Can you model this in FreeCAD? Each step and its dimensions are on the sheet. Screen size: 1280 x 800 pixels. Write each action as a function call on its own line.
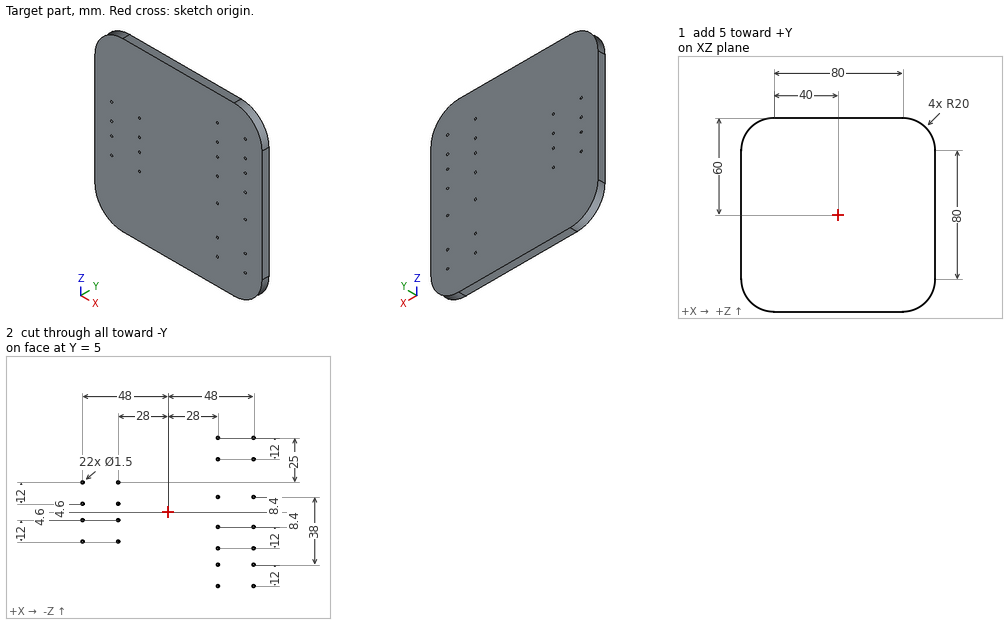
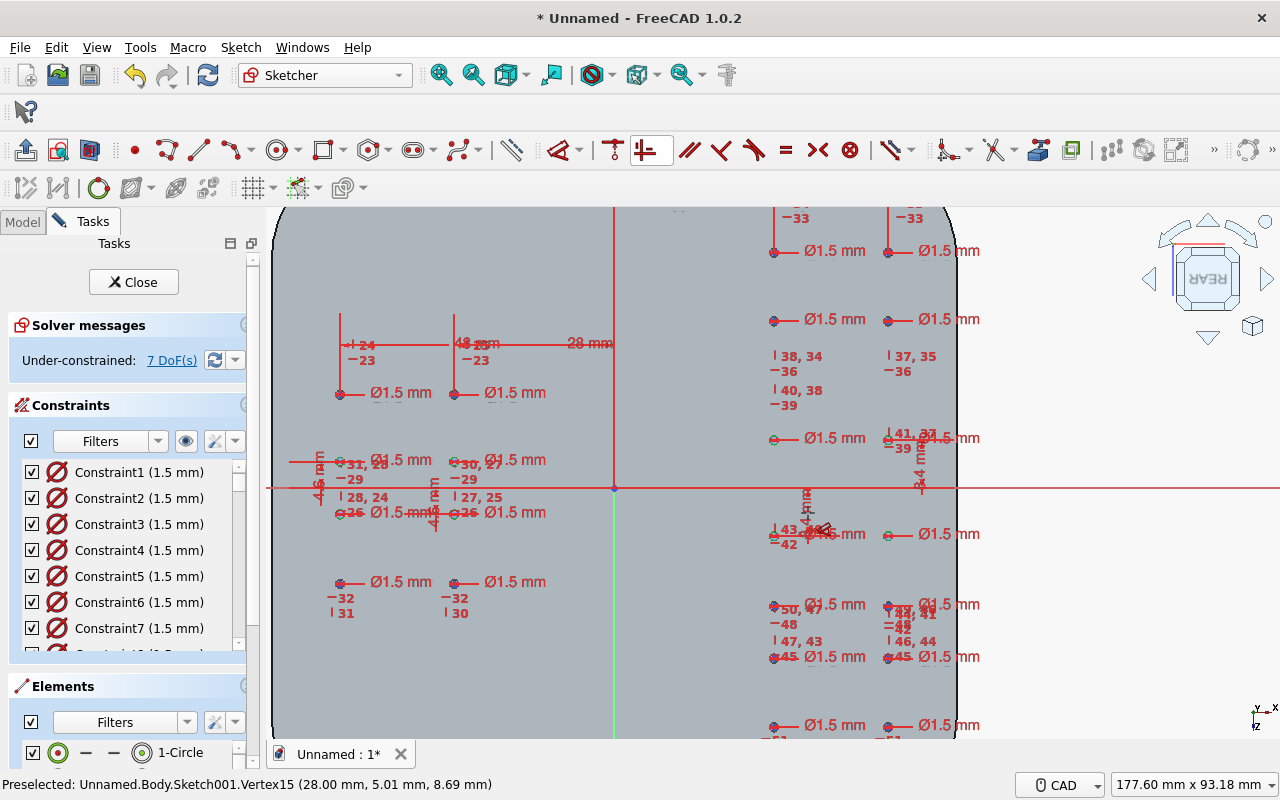
click(340, 395)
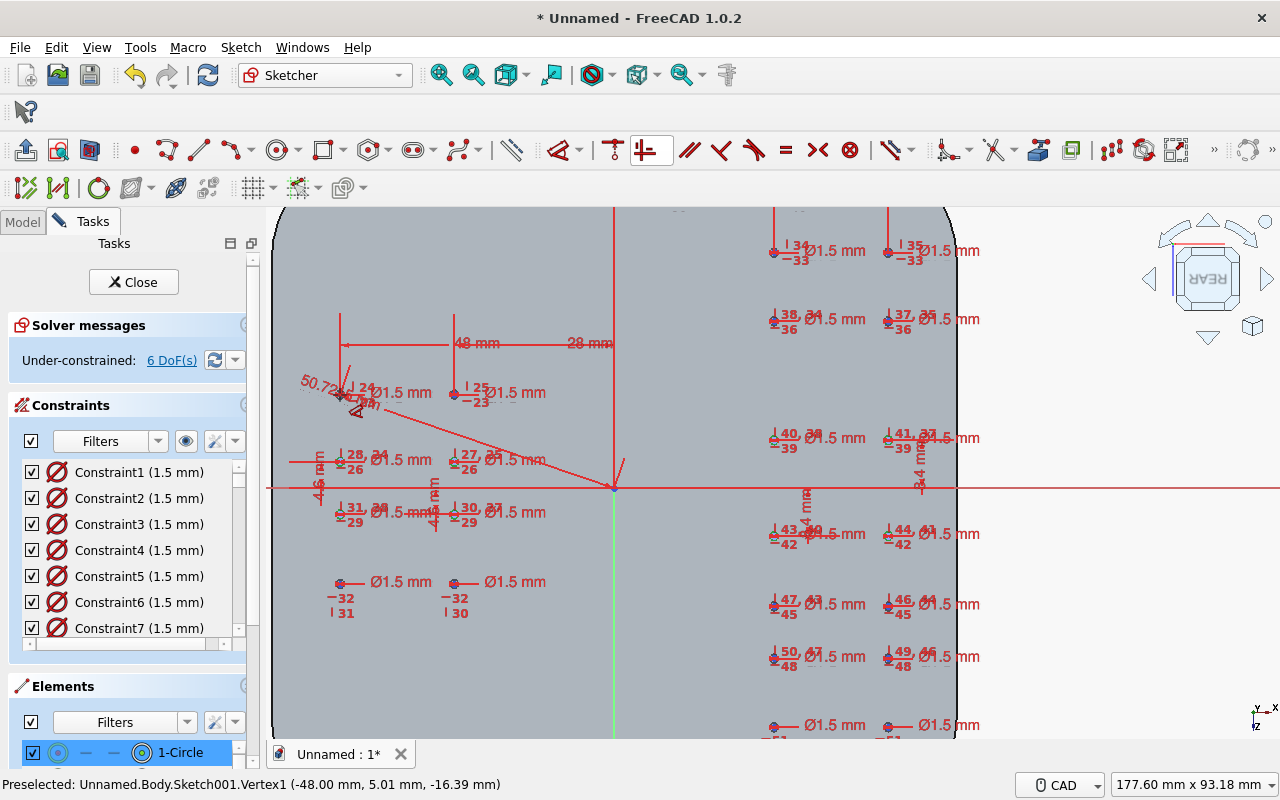
click(340, 462)
click(306, 428)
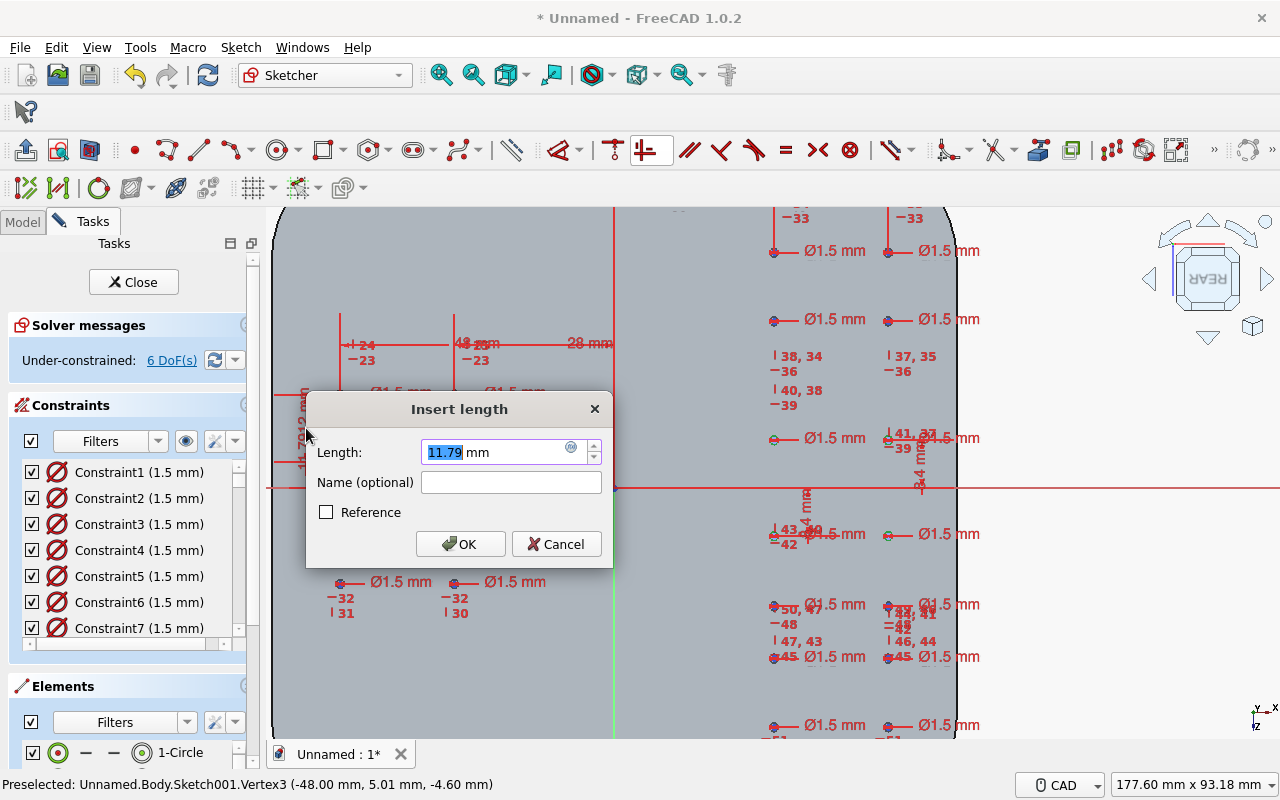
text(12)
key(Return)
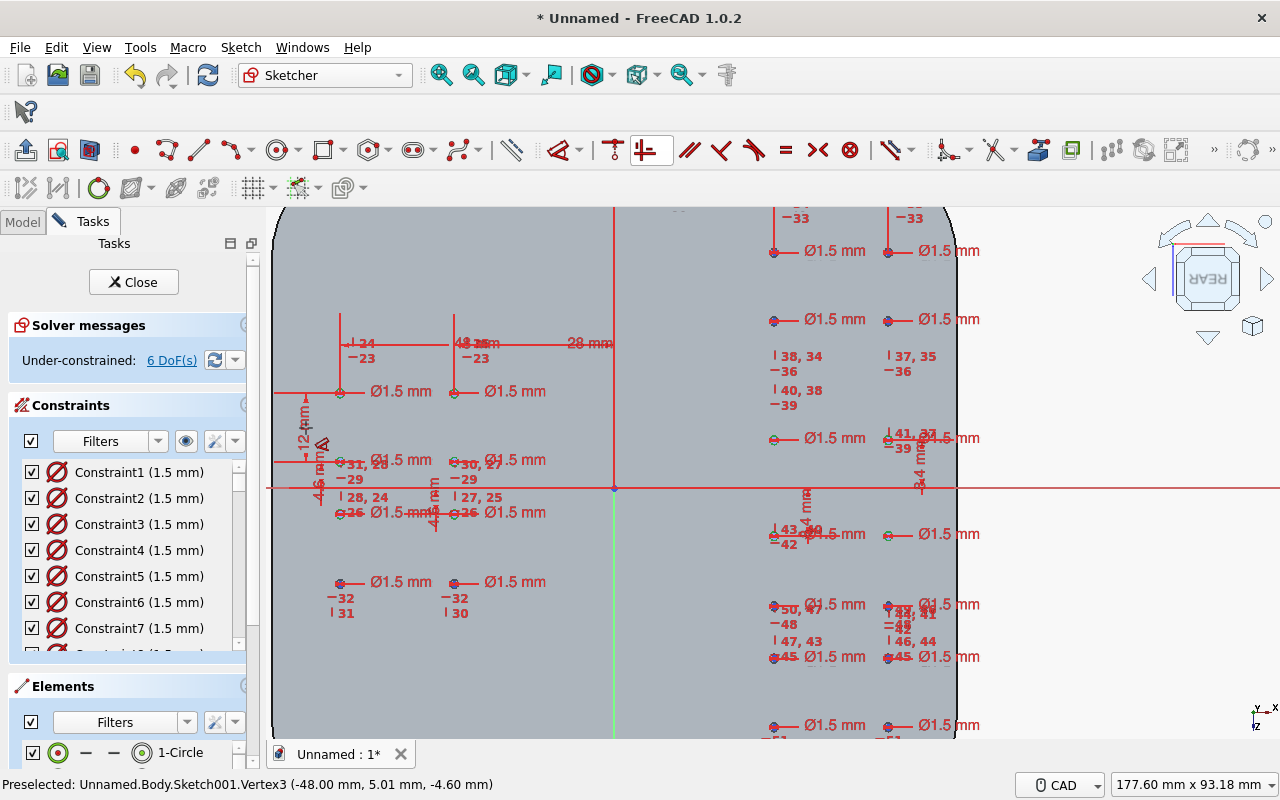
click(454, 514)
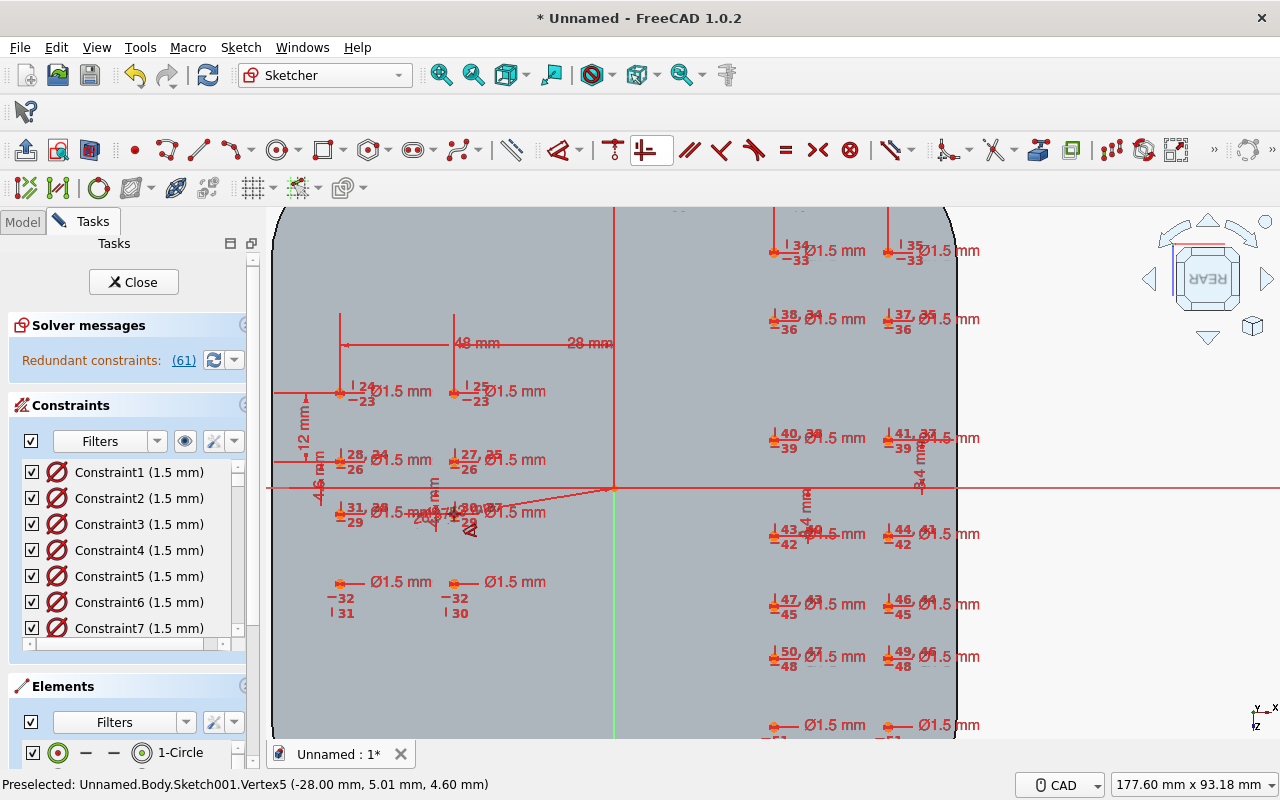
click(454, 584)
click(420, 549)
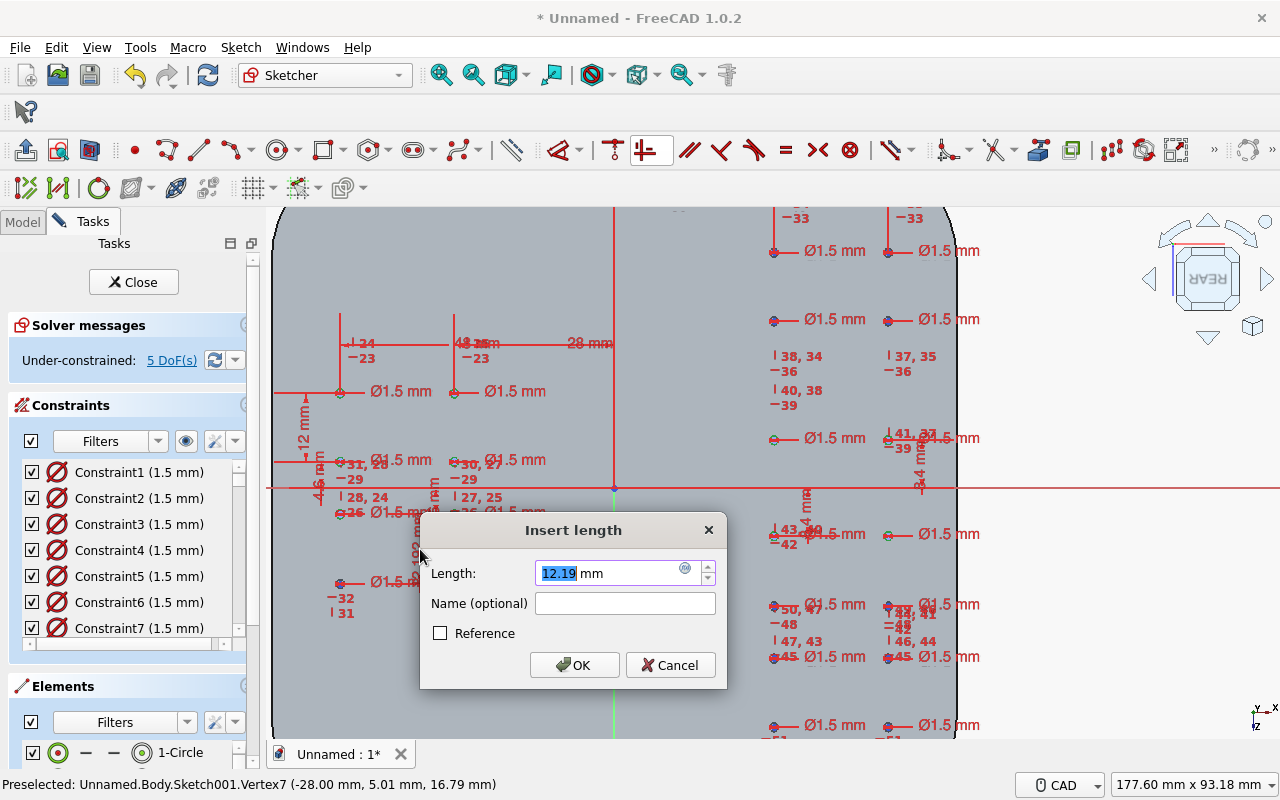
text(12)
key(Return)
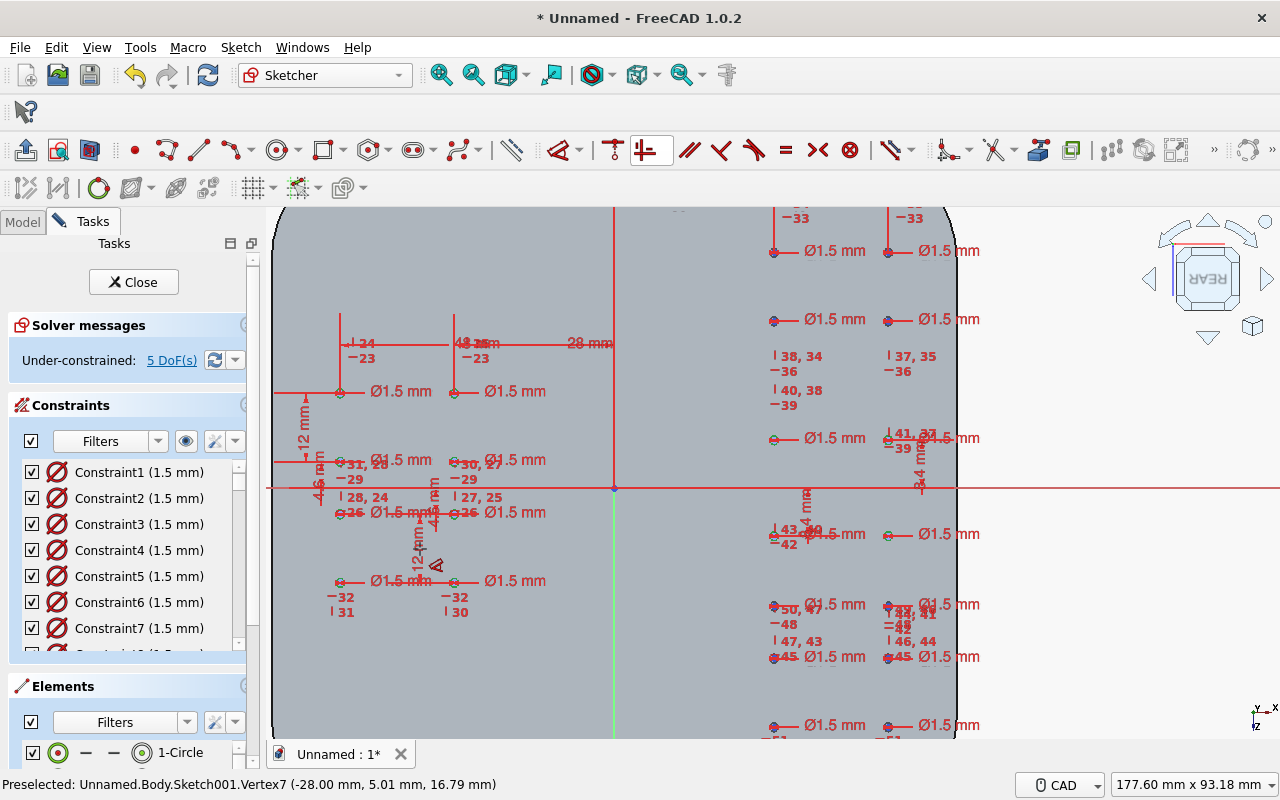
click(454, 393)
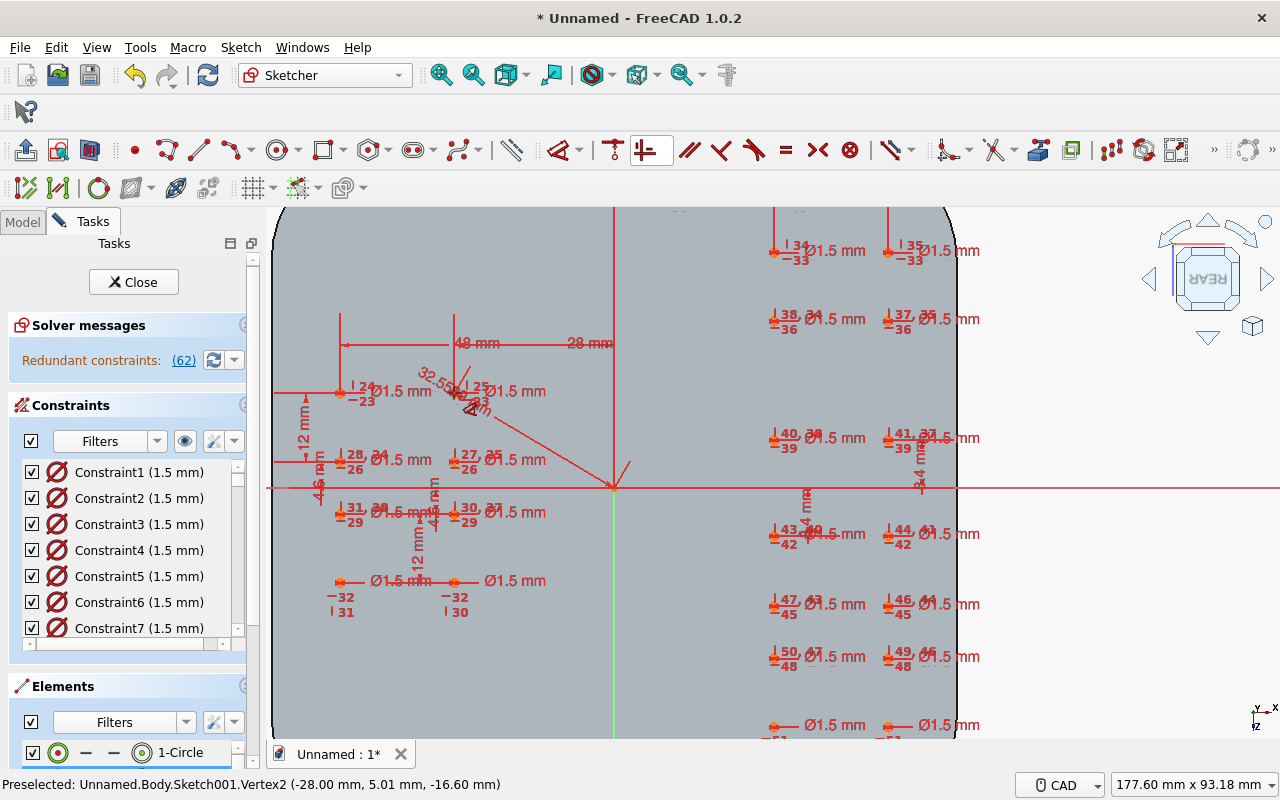
click(774, 253)
click(808, 323)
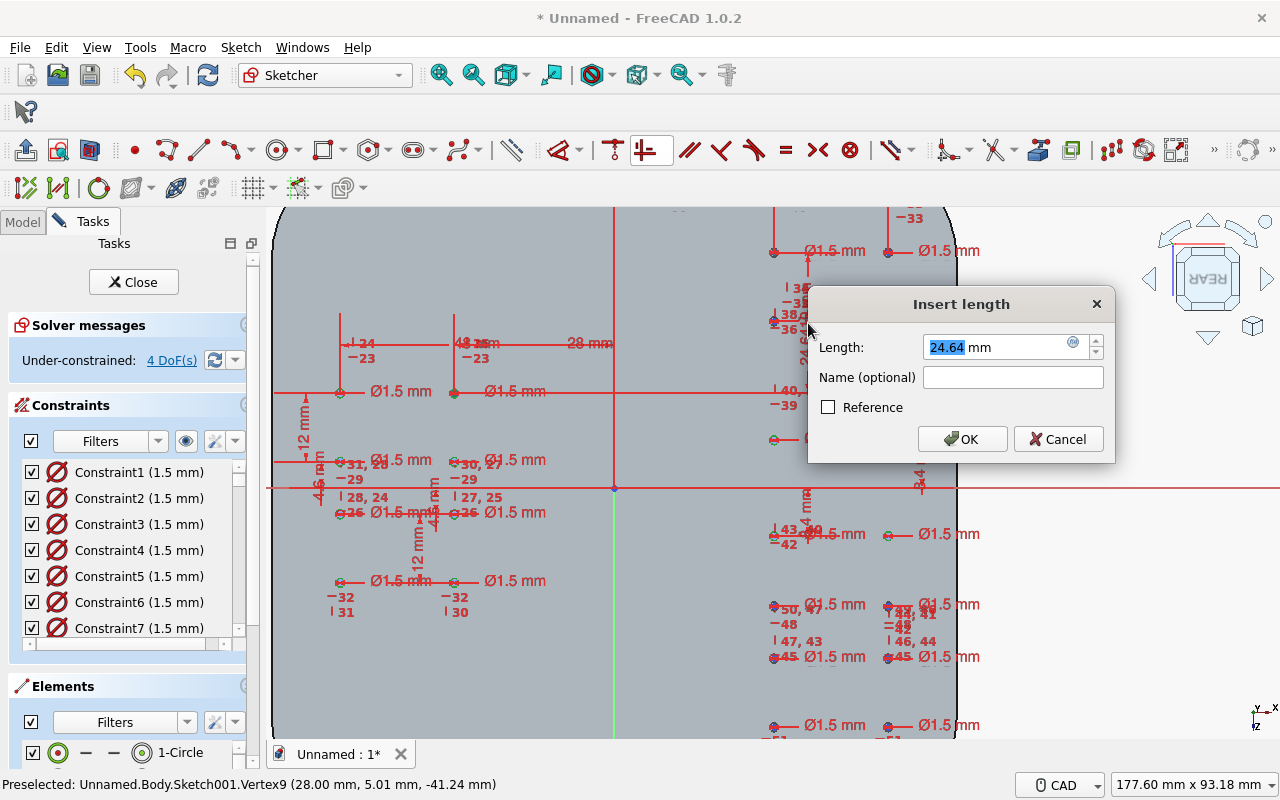
text(25)
key(Return)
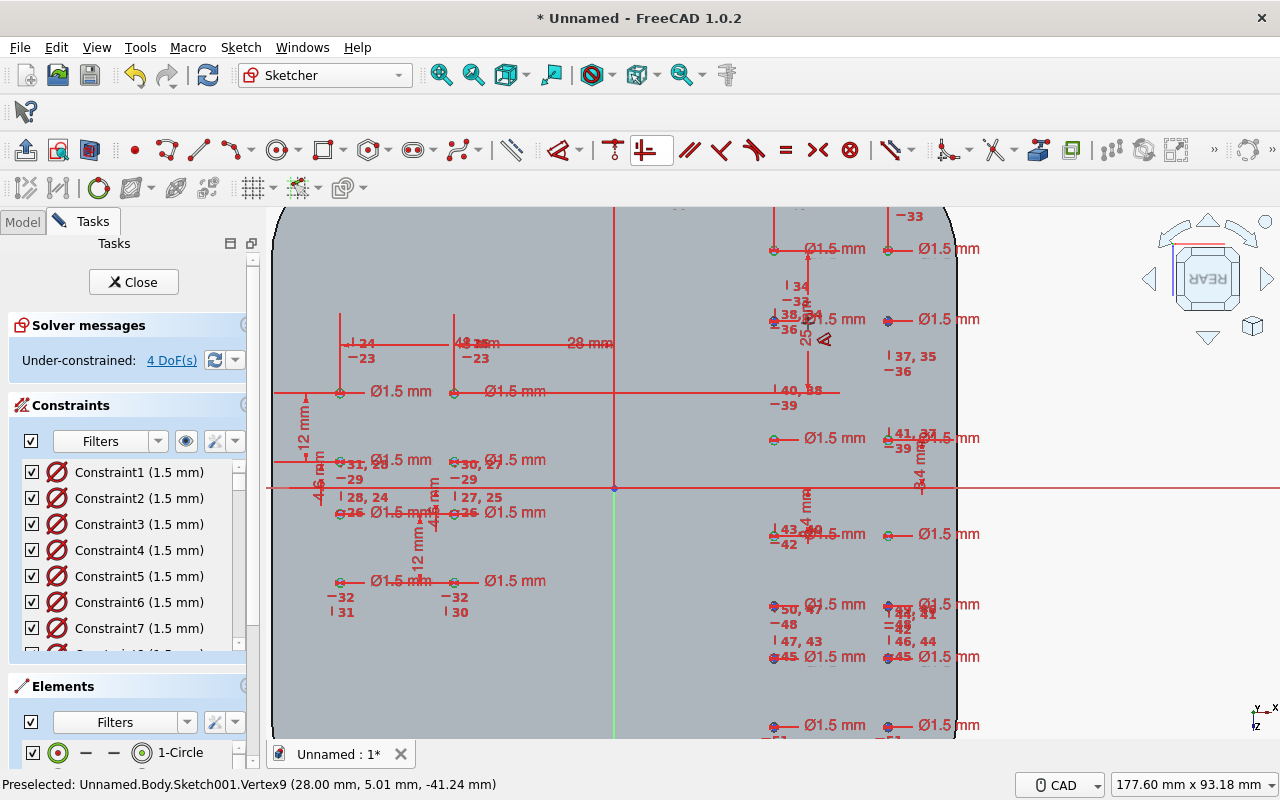
click(774, 251)